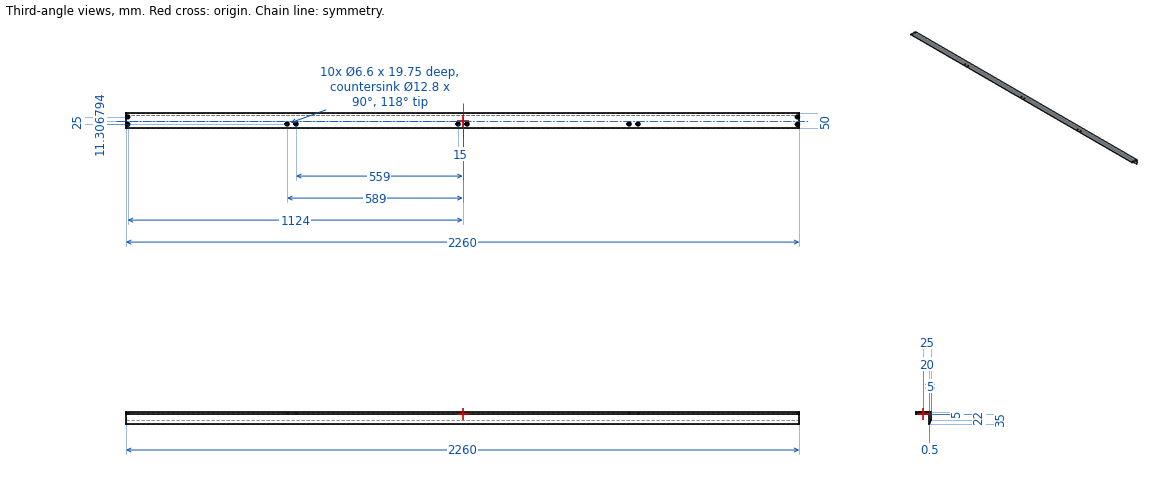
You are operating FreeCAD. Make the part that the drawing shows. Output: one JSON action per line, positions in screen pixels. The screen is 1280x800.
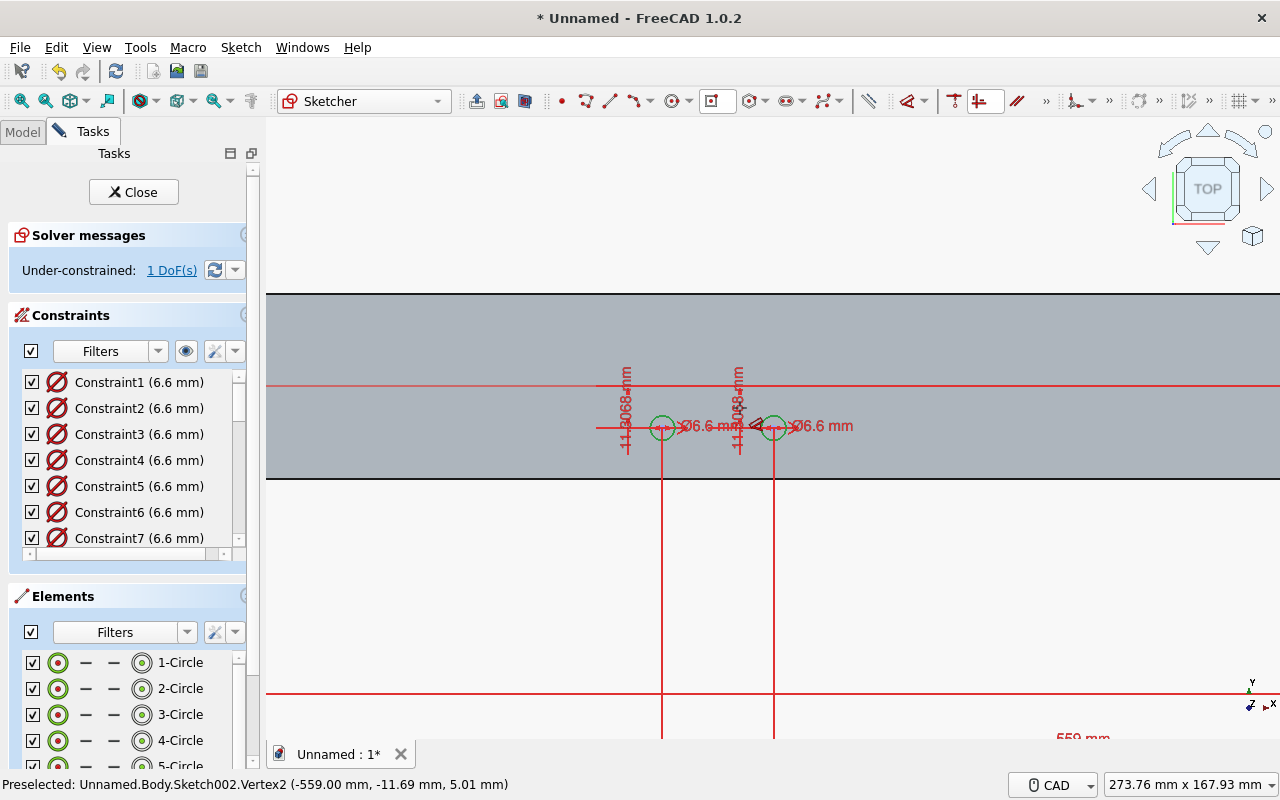
{"action": "scroll", "coordinate": [533, 431], "scroll_direction": "down", "scroll_amount": 13}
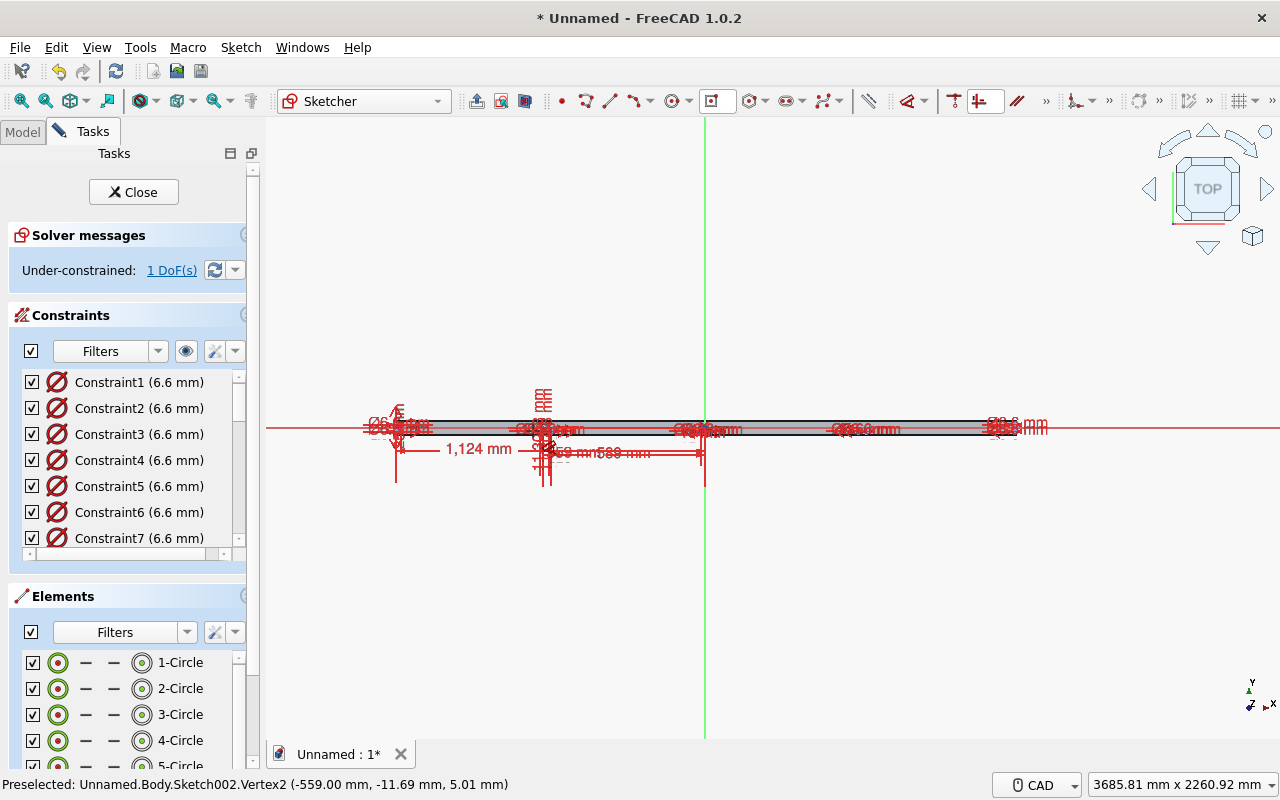
{"action": "scroll", "coordinate": [701, 431], "scroll_direction": "up", "scroll_amount": 13}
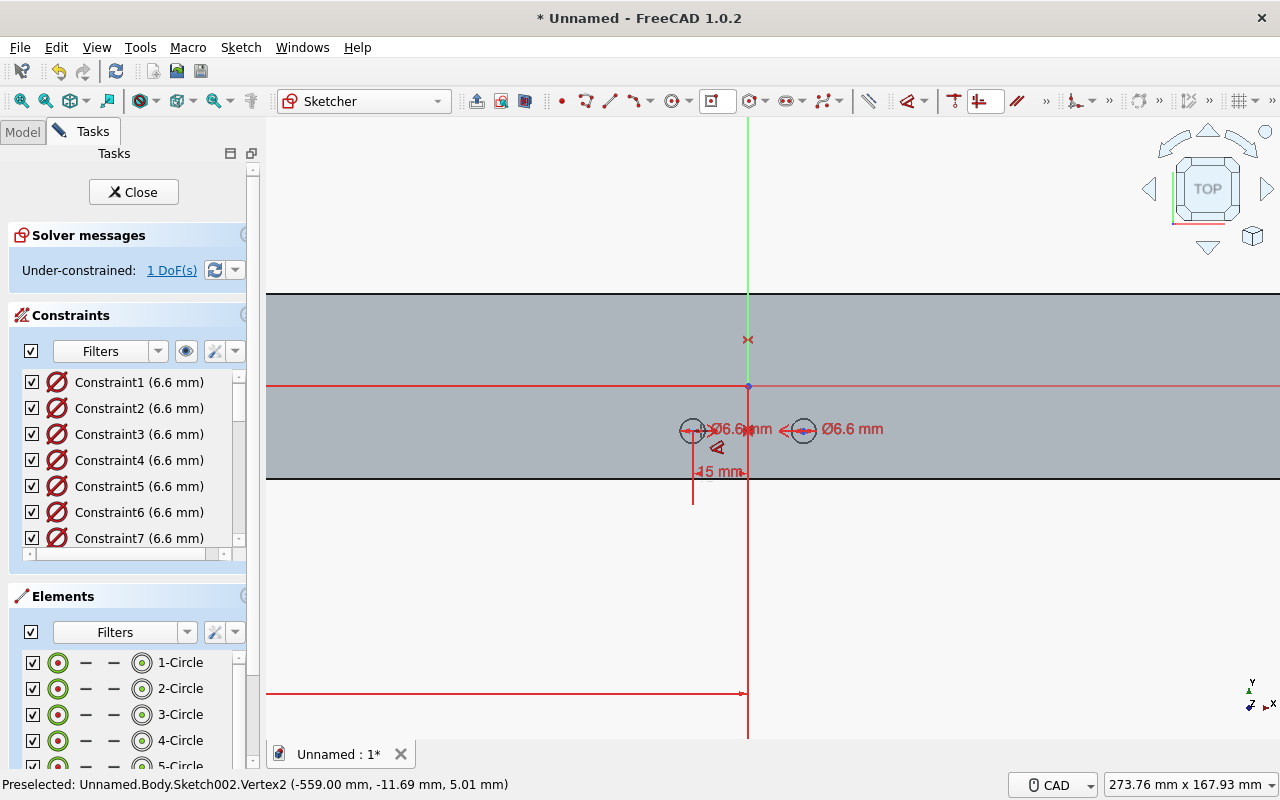
{"action": "left_click", "coordinate": [693, 431]}
{"action": "left_click", "coordinate": [659, 409]}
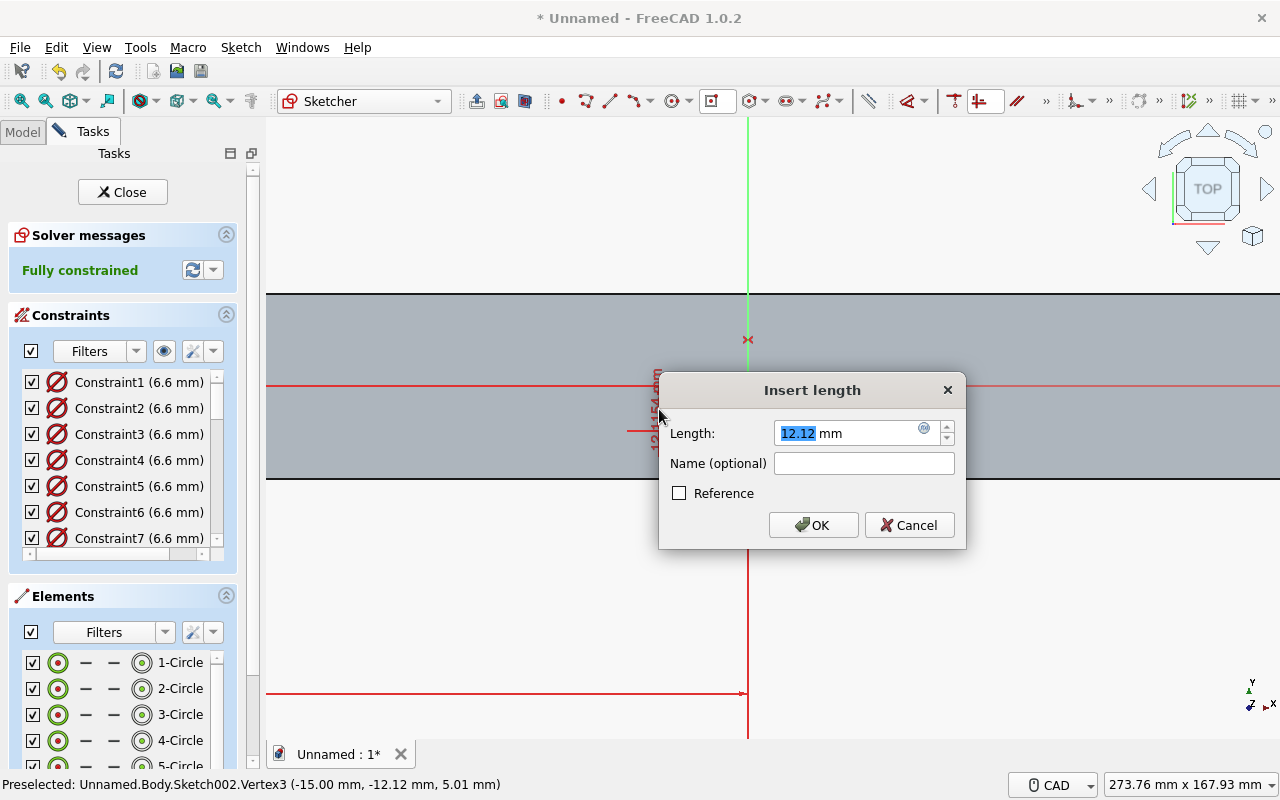
{"action": "type", "text": "11.306794"}
{"action": "key", "text": "Return"}
{"action": "key", "text": "Escape"}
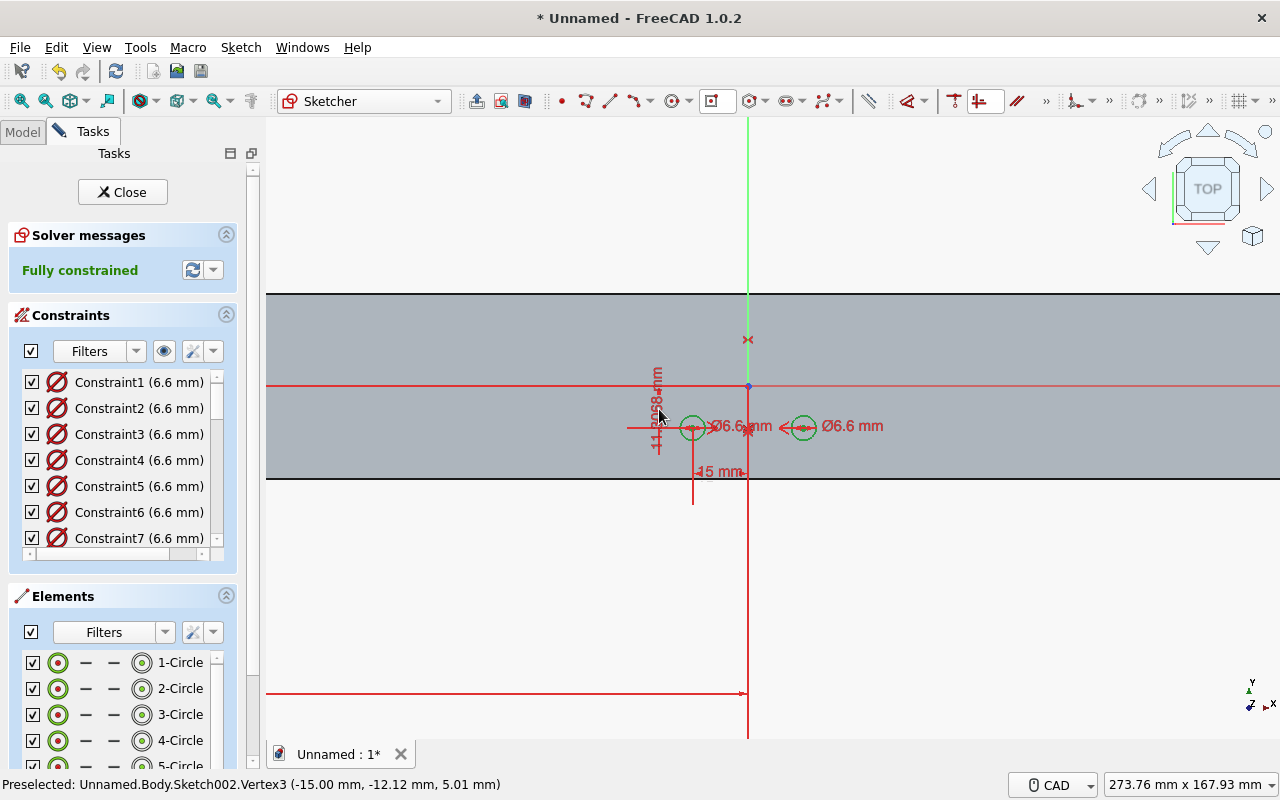
{"action": "left_click", "coordinate": [123, 192]}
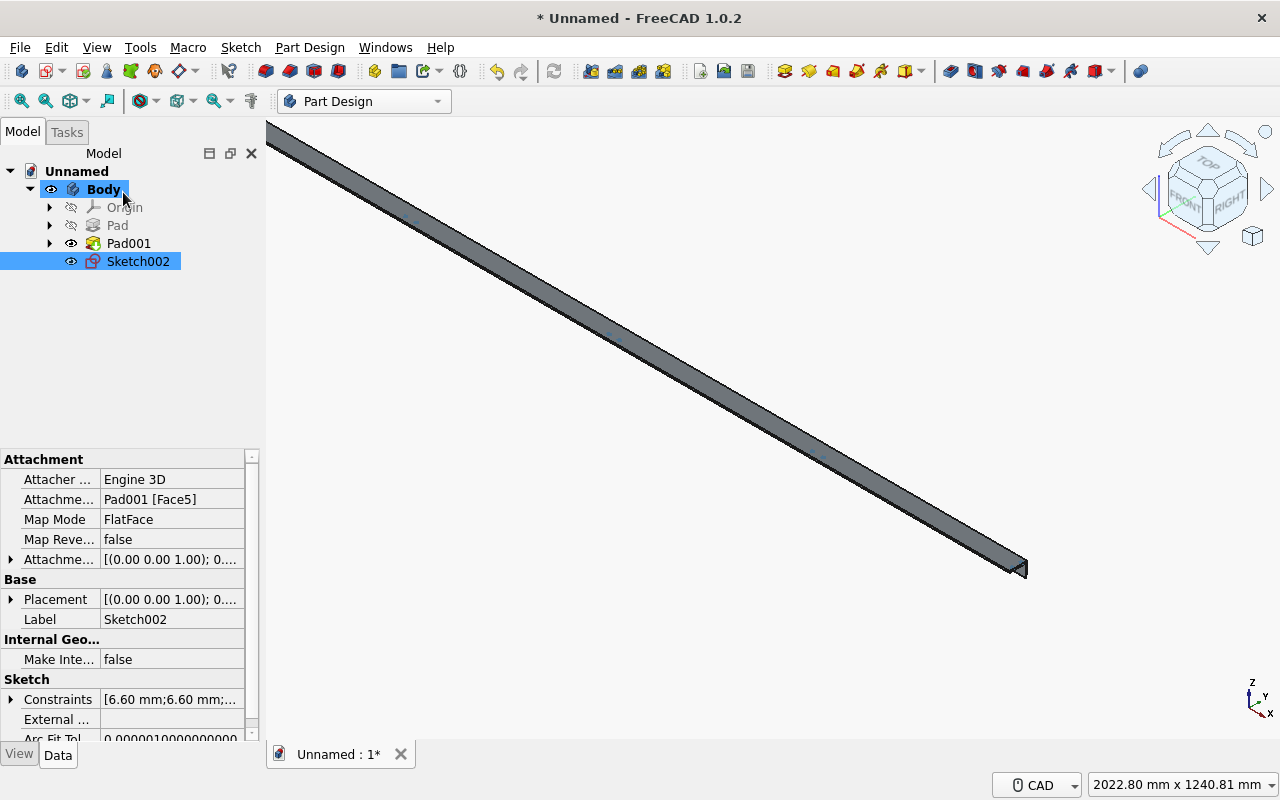
{"action": "left_click", "coordinate": [976, 72]}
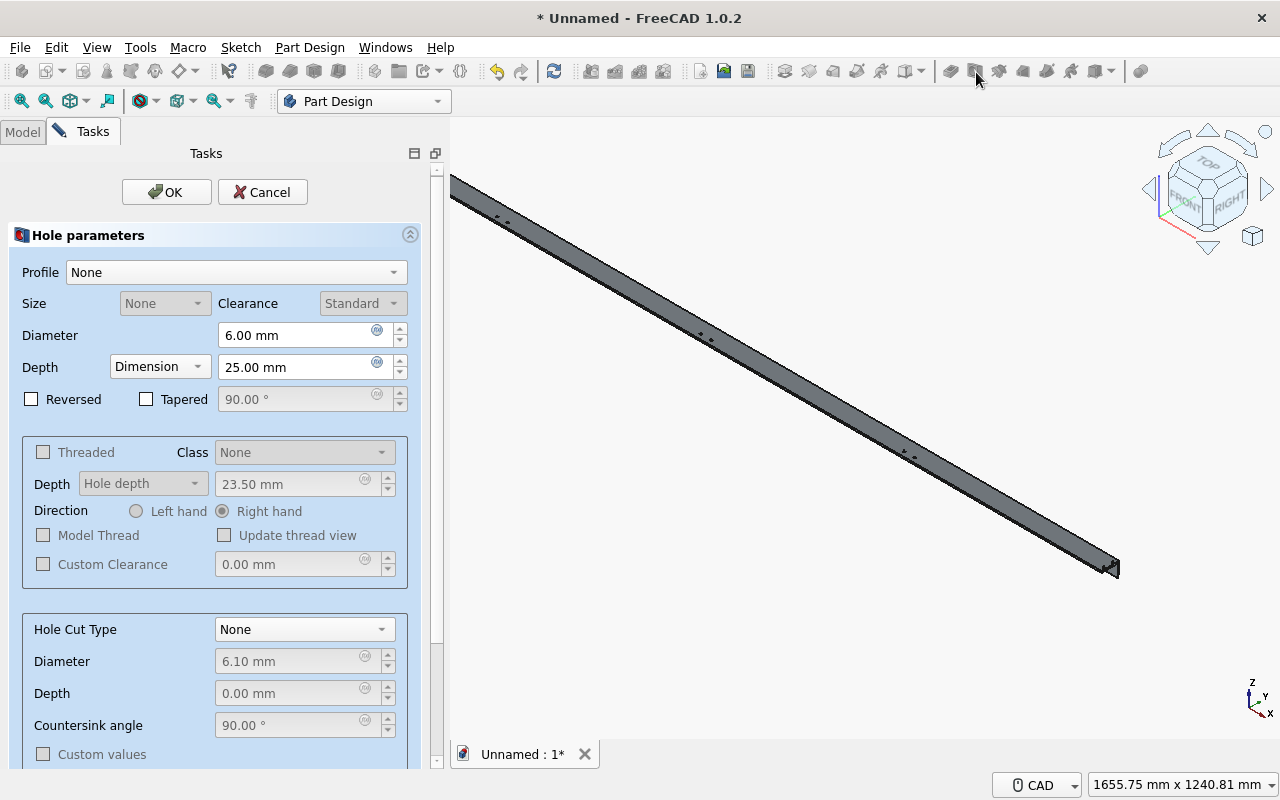
{"action": "triple_click", "coordinate": [305, 335]}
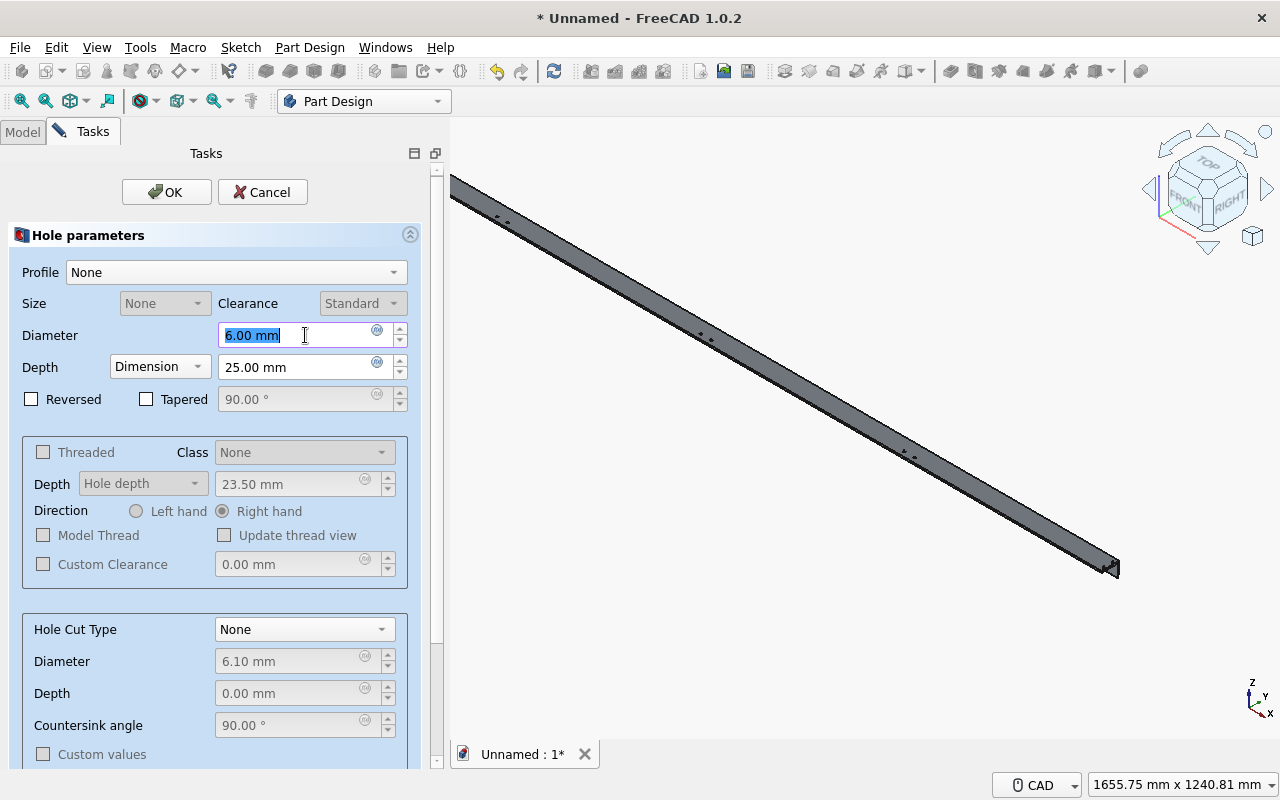
{"action": "type", "text": "6.6"}
{"action": "key", "text": "Tab"}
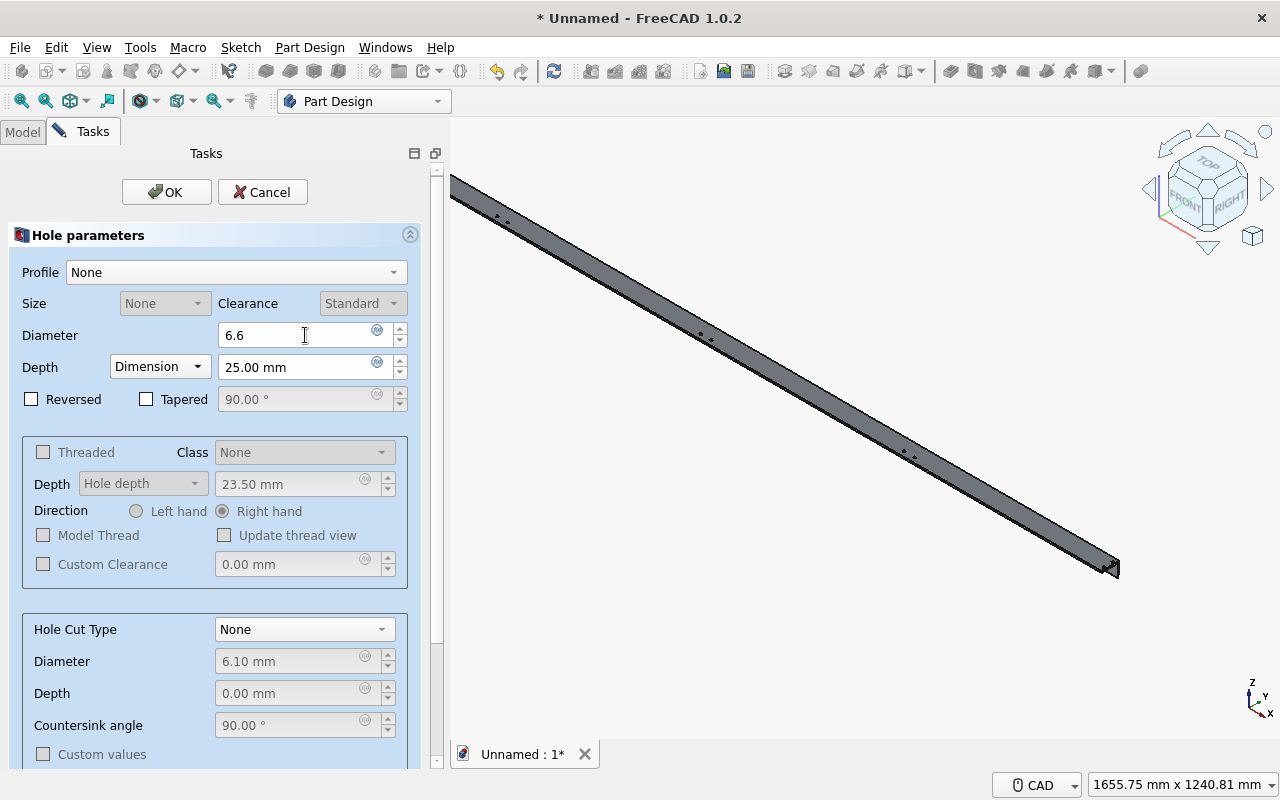
{"action": "triple_click", "coordinate": [305, 367]}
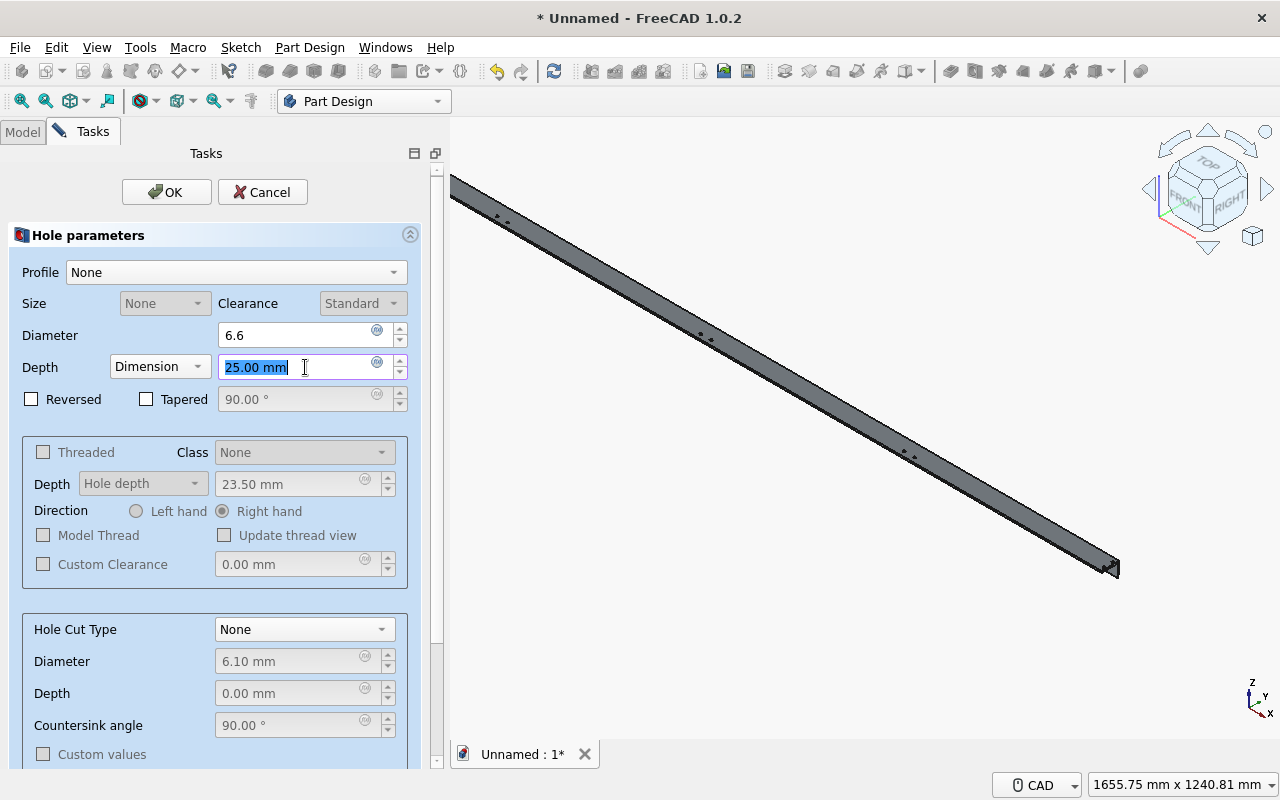
{"action": "type", "text": "19.75"}
{"action": "key", "text": "Tab"}